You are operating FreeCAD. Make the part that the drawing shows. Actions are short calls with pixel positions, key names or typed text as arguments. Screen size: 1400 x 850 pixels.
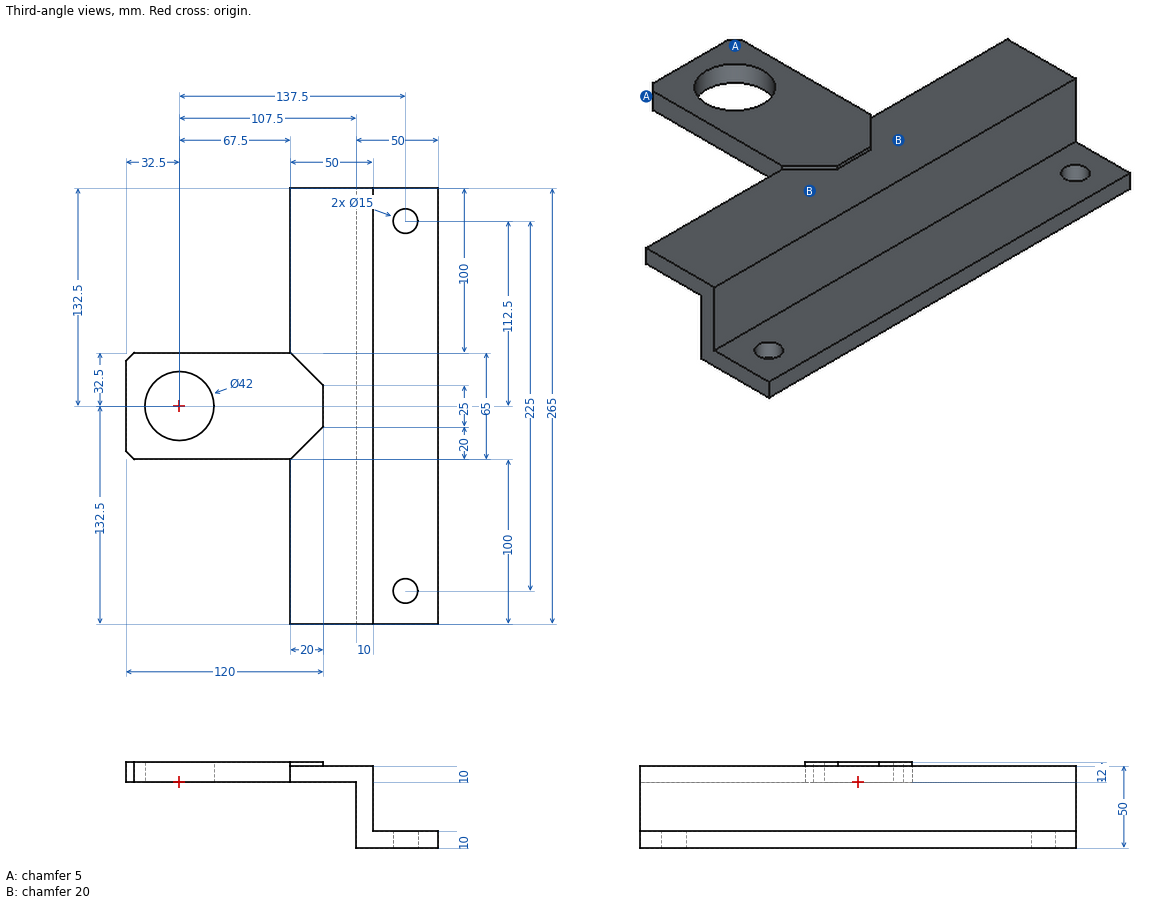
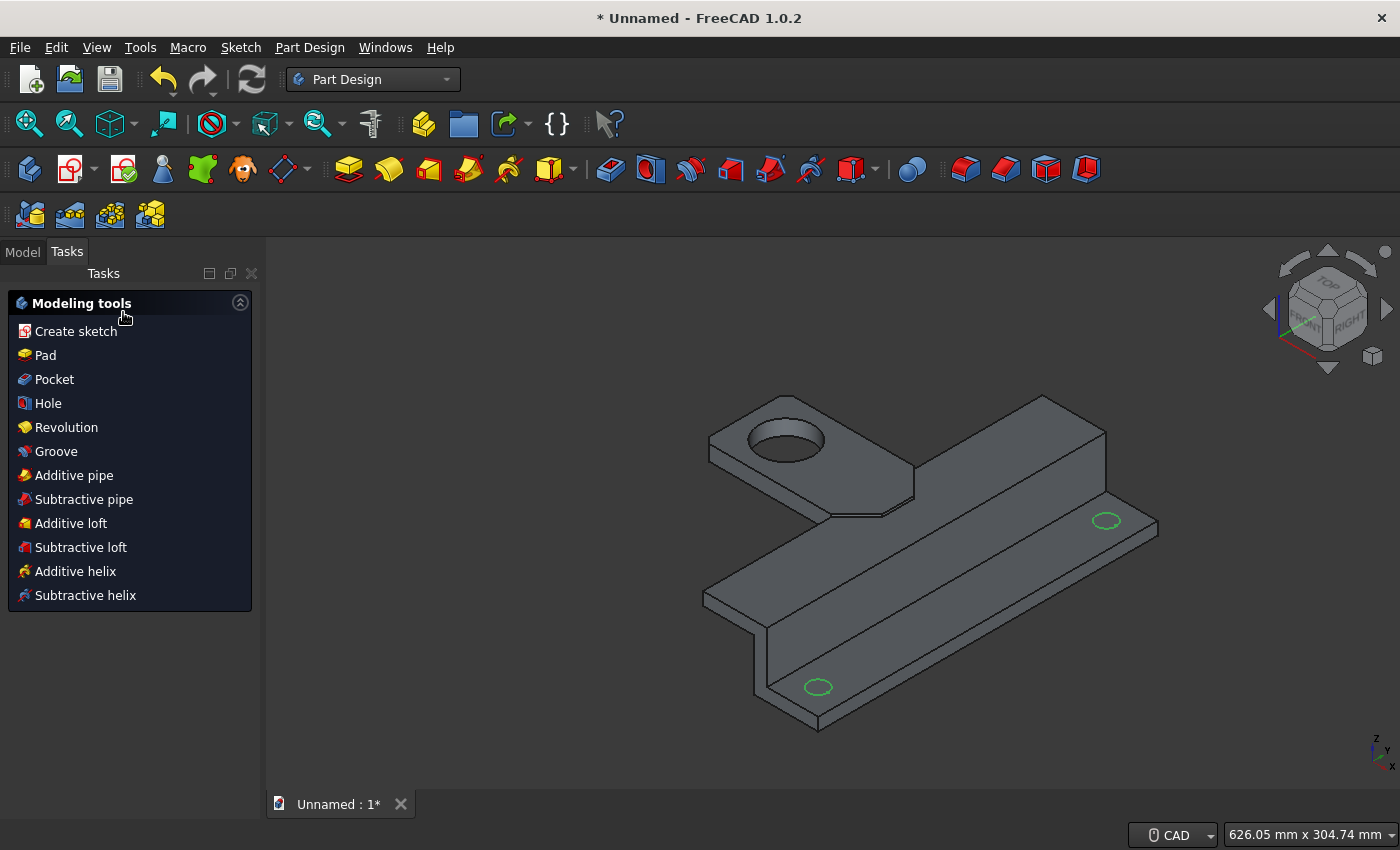
click(612, 170)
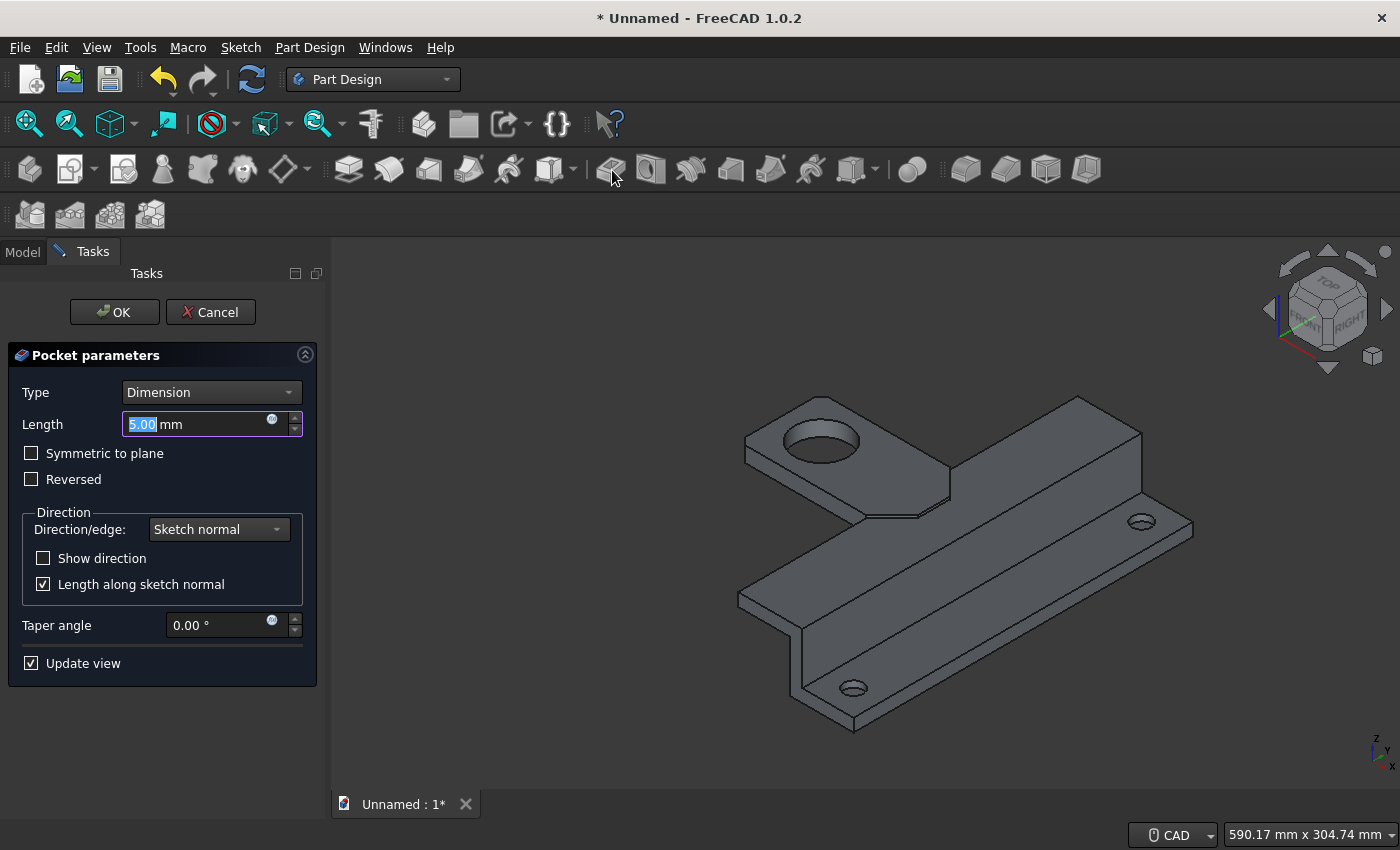
click(212, 392)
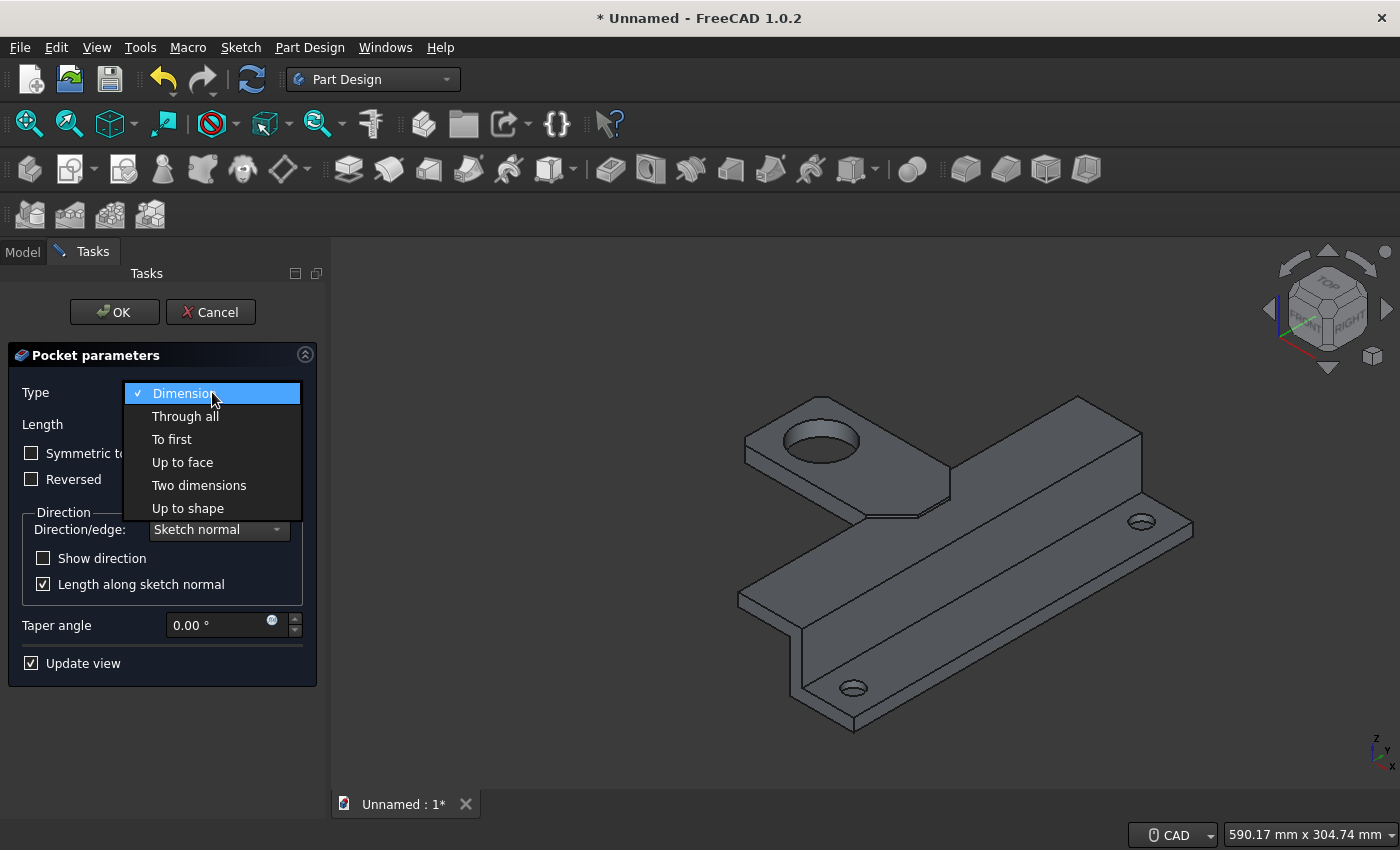
click(212, 416)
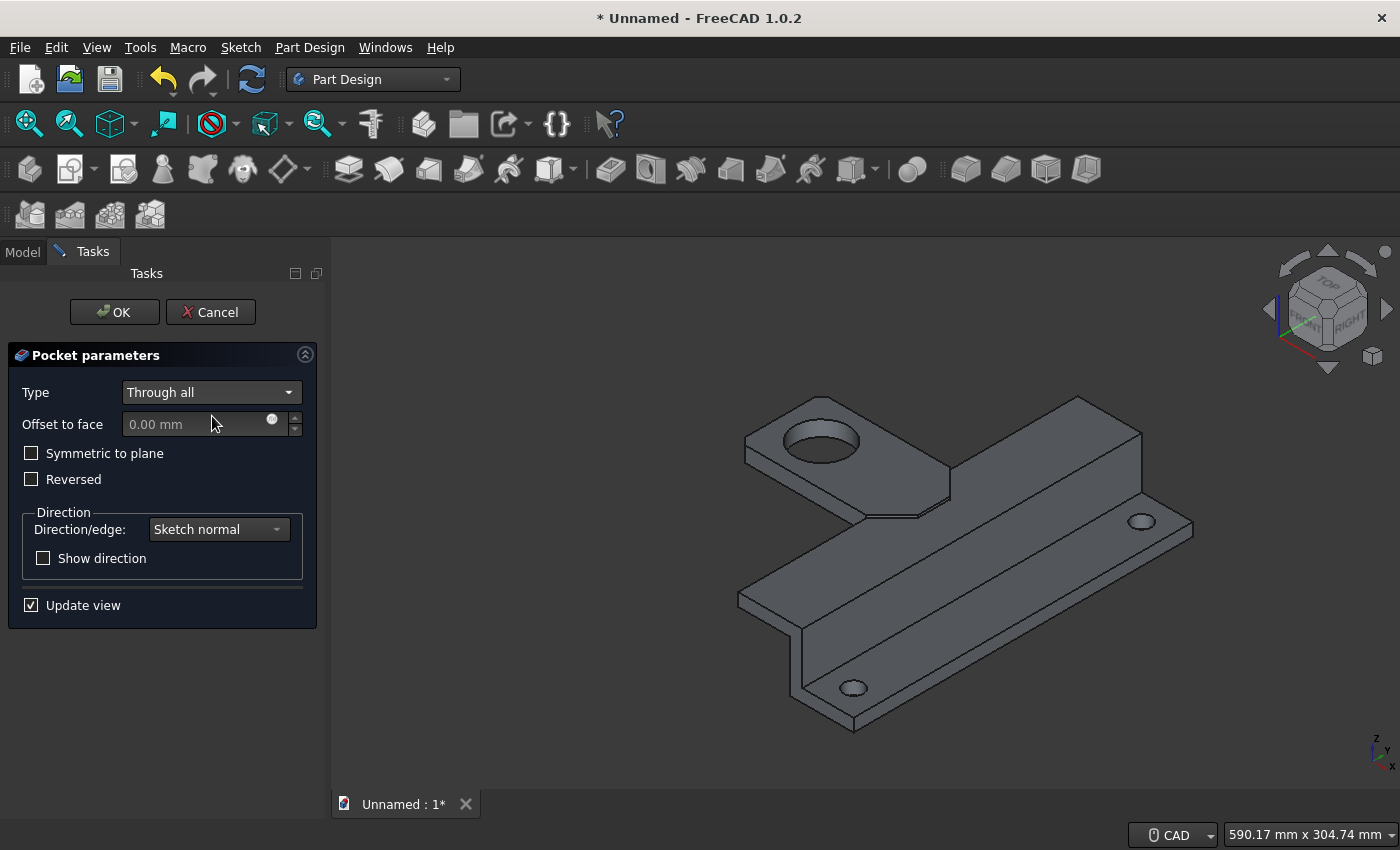
click(115, 312)